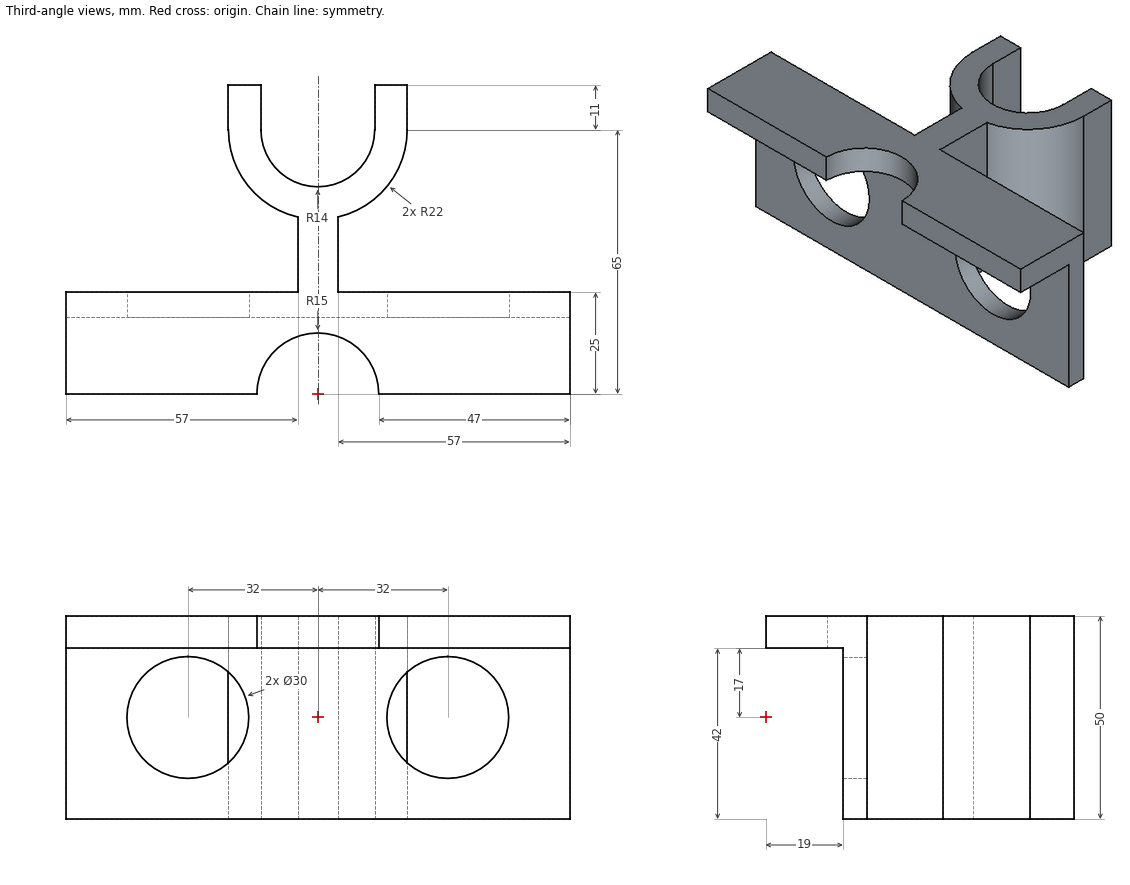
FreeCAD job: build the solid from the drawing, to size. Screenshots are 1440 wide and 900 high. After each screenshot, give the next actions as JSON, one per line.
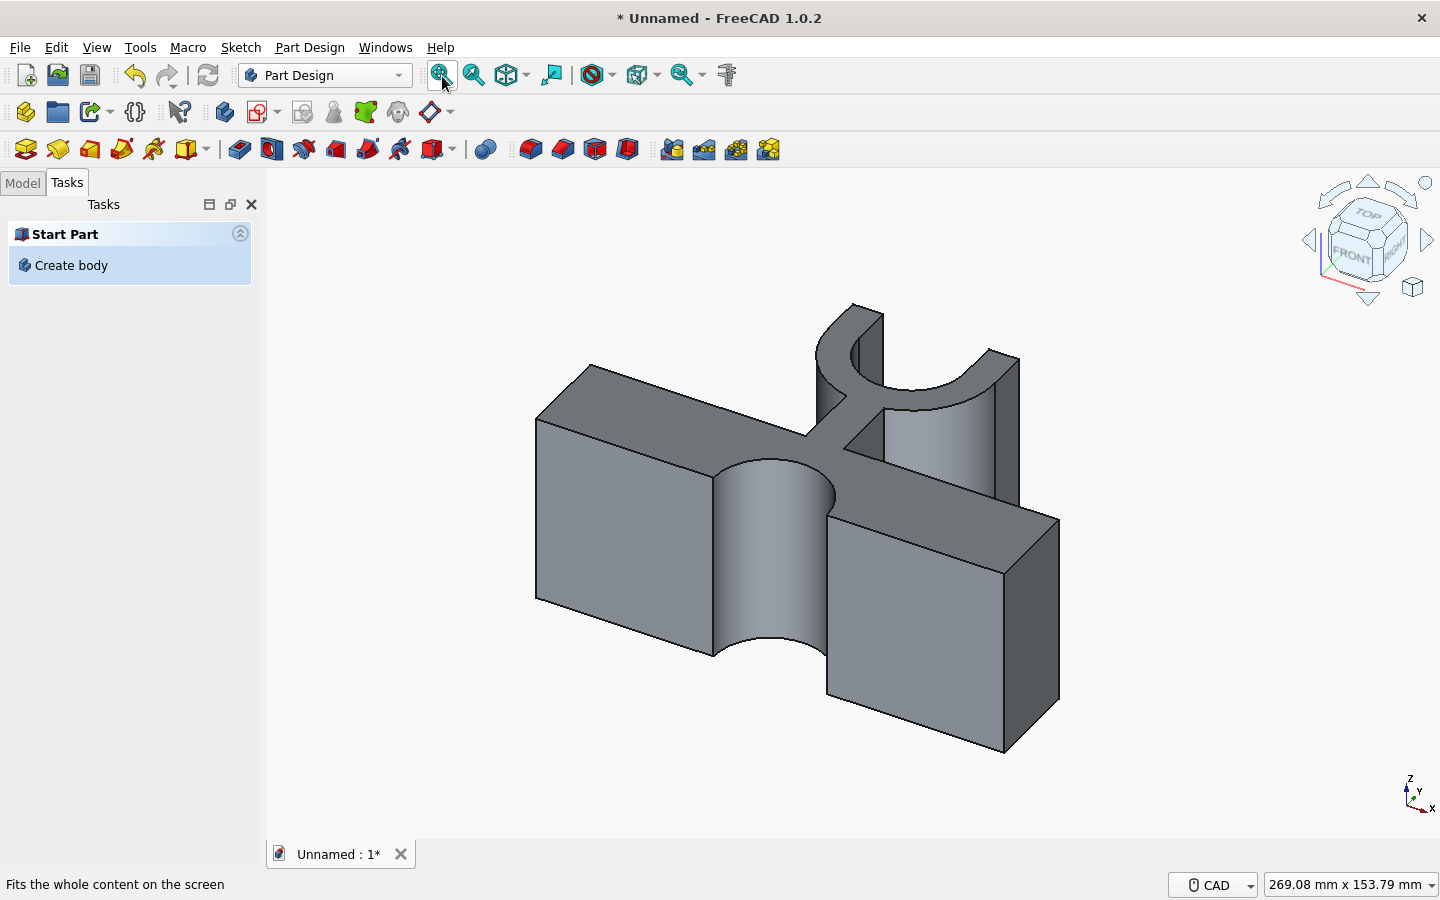
{"action": "left_click", "coordinate": [1032, 610]}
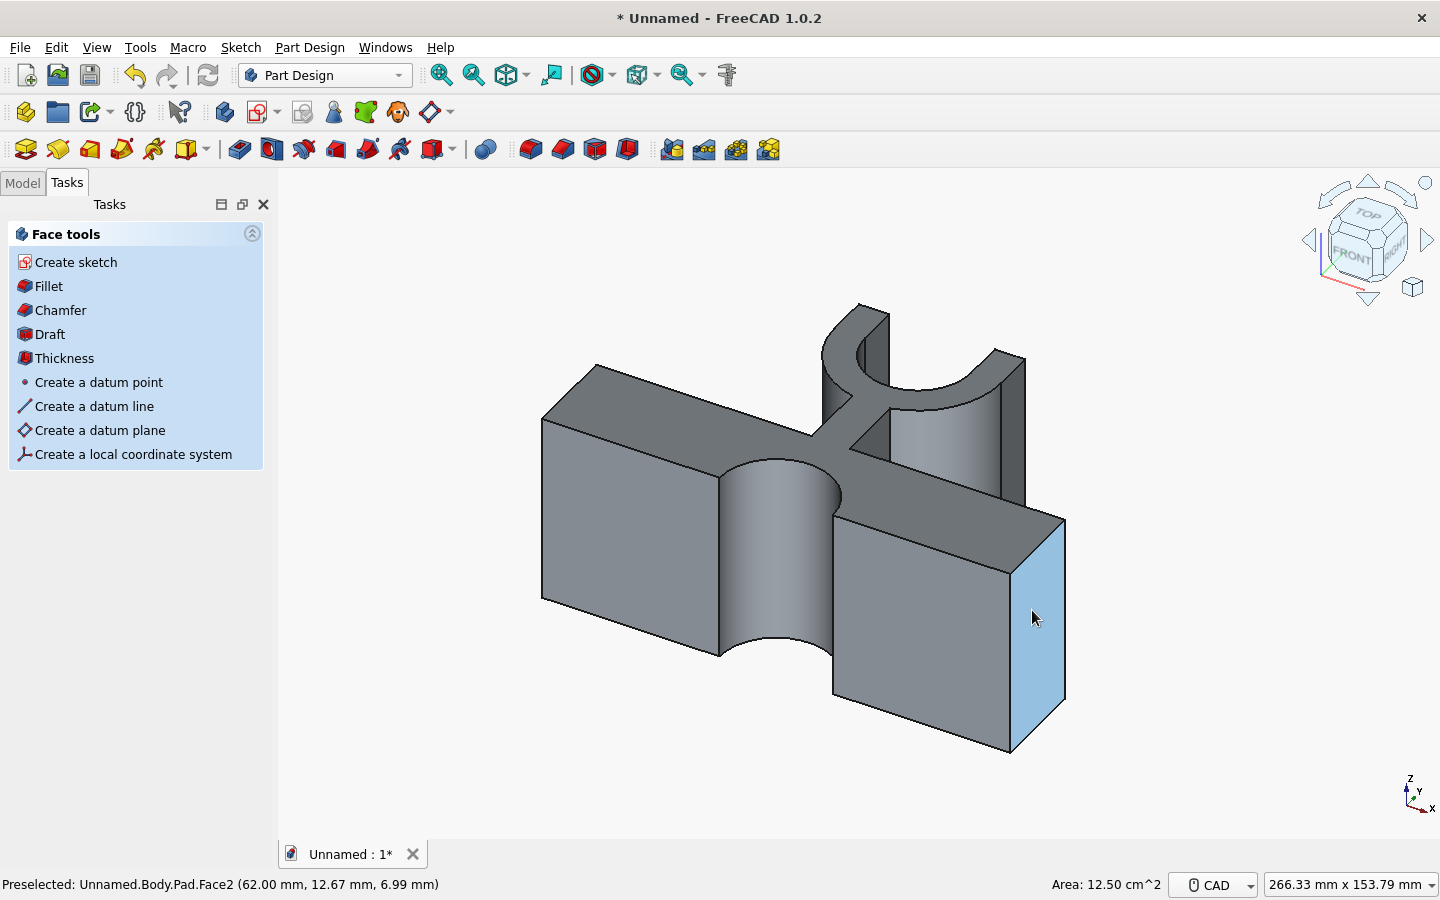
{"action": "left_click", "coordinate": [258, 112]}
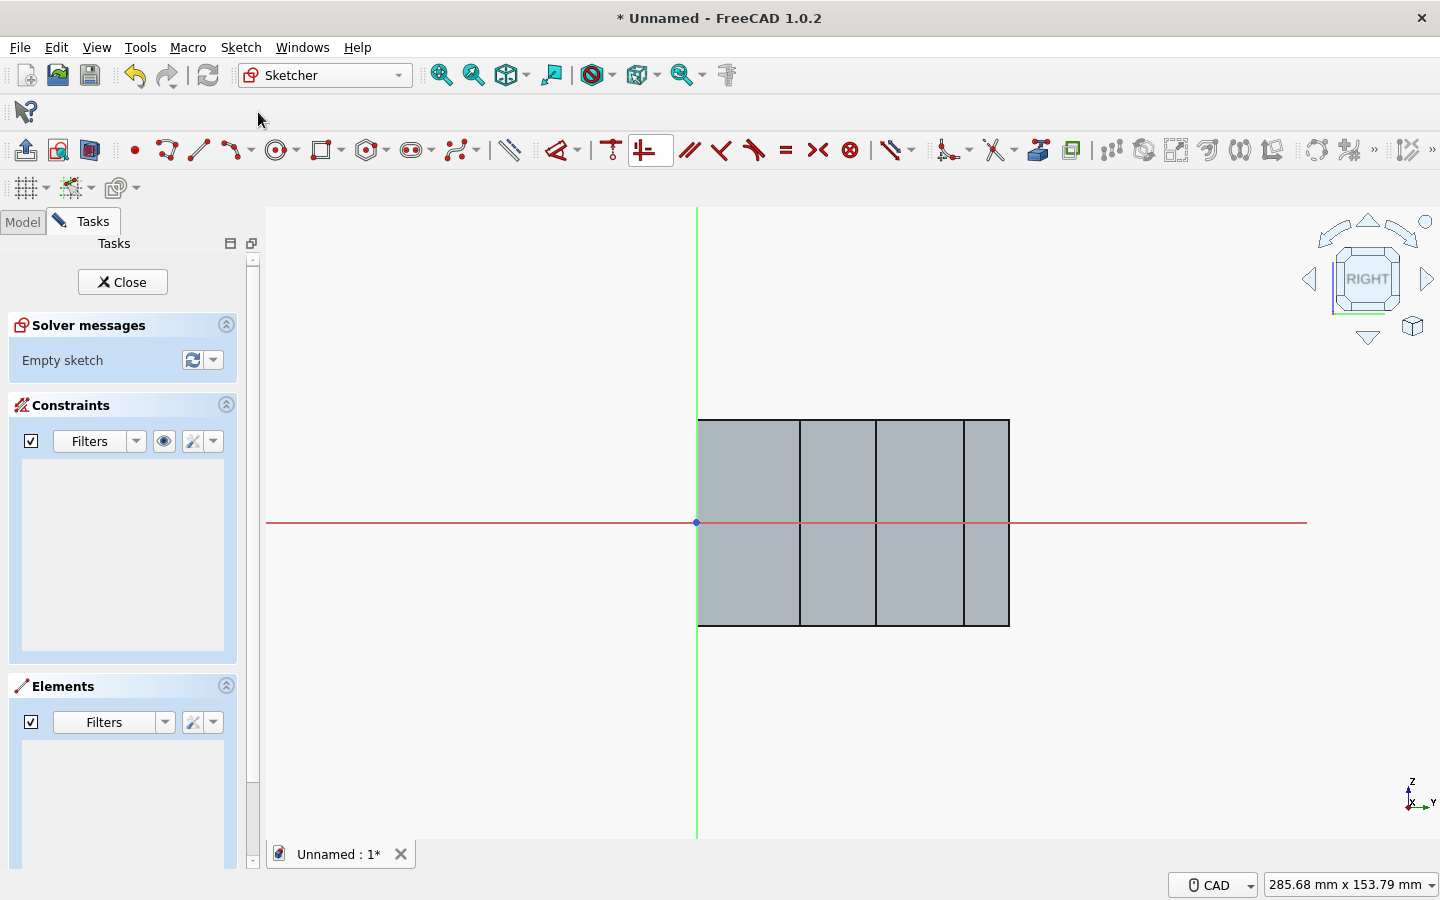
{"action": "scroll", "coordinate": [696, 553], "scroll_direction": "up", "scroll_amount": 4}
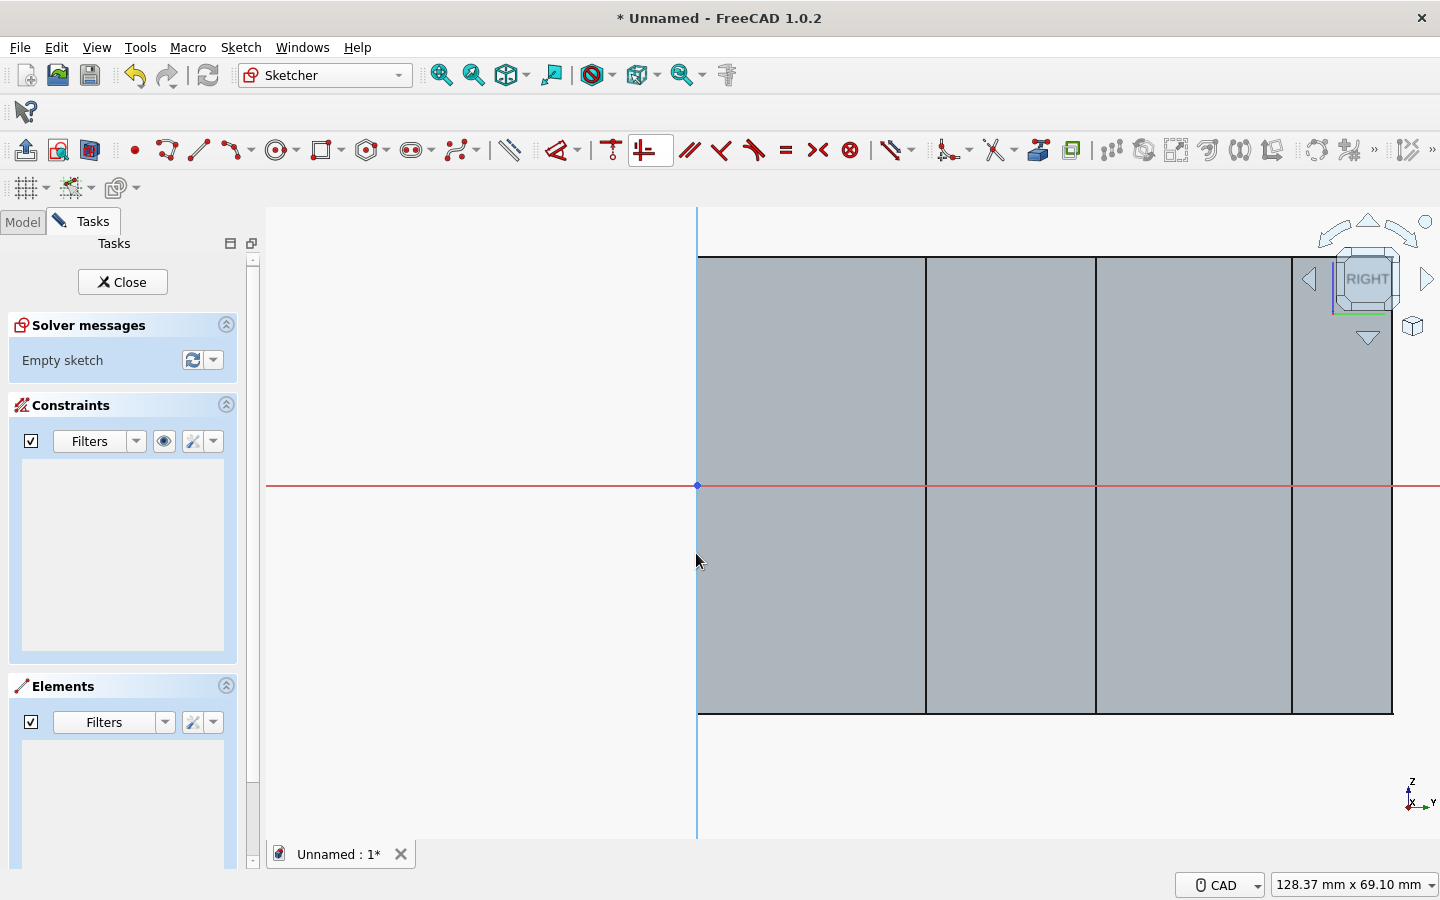
{"action": "left_click", "coordinate": [322, 150]}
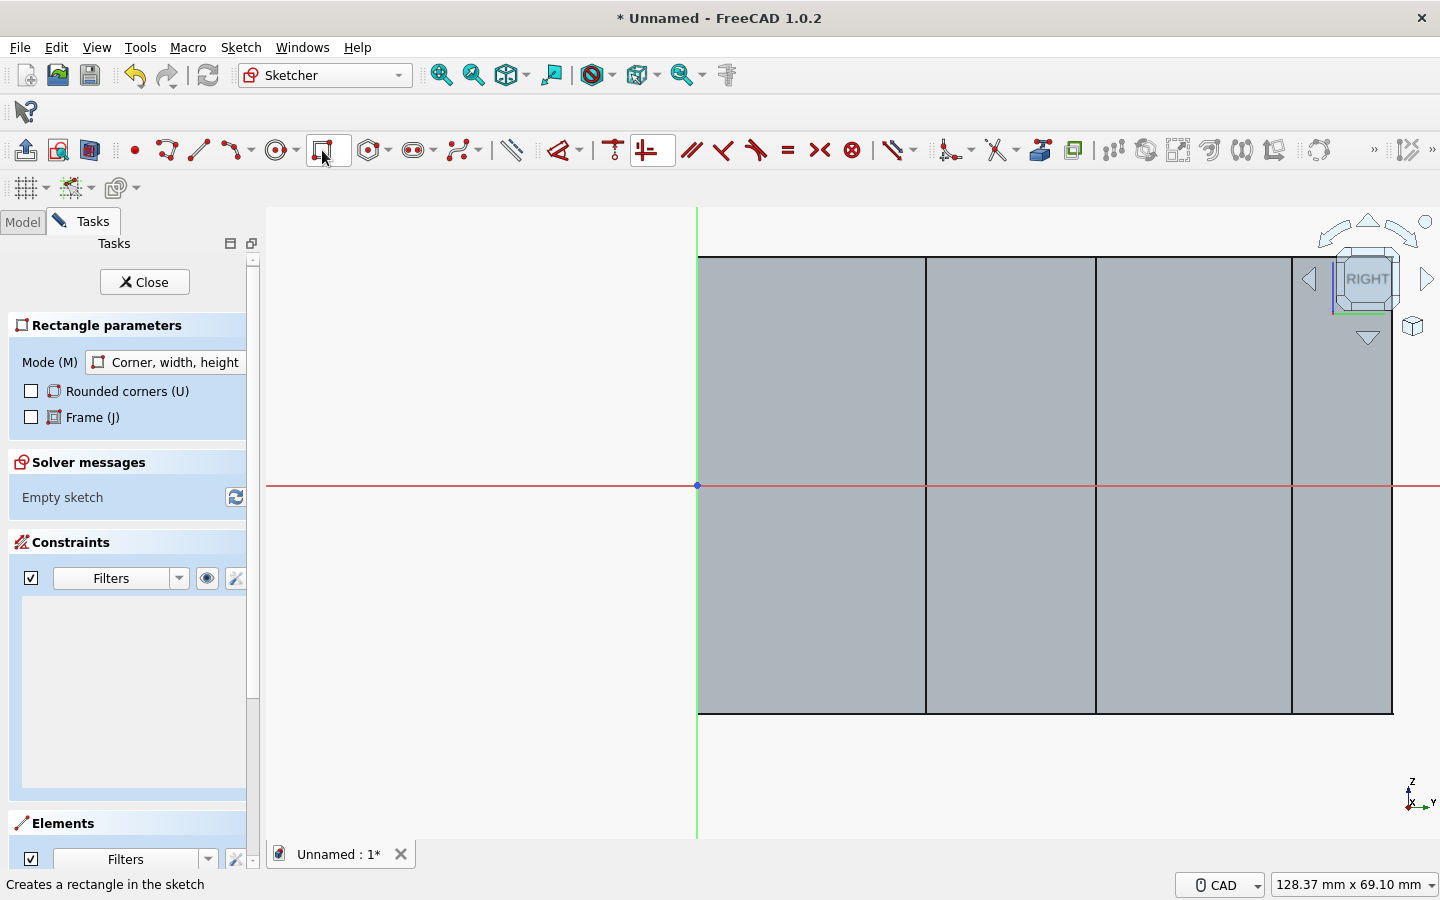
{"action": "left_click", "coordinate": [697, 330]}
{"action": "left_click", "coordinate": [871, 714]}
{"action": "key", "text": "Escape"}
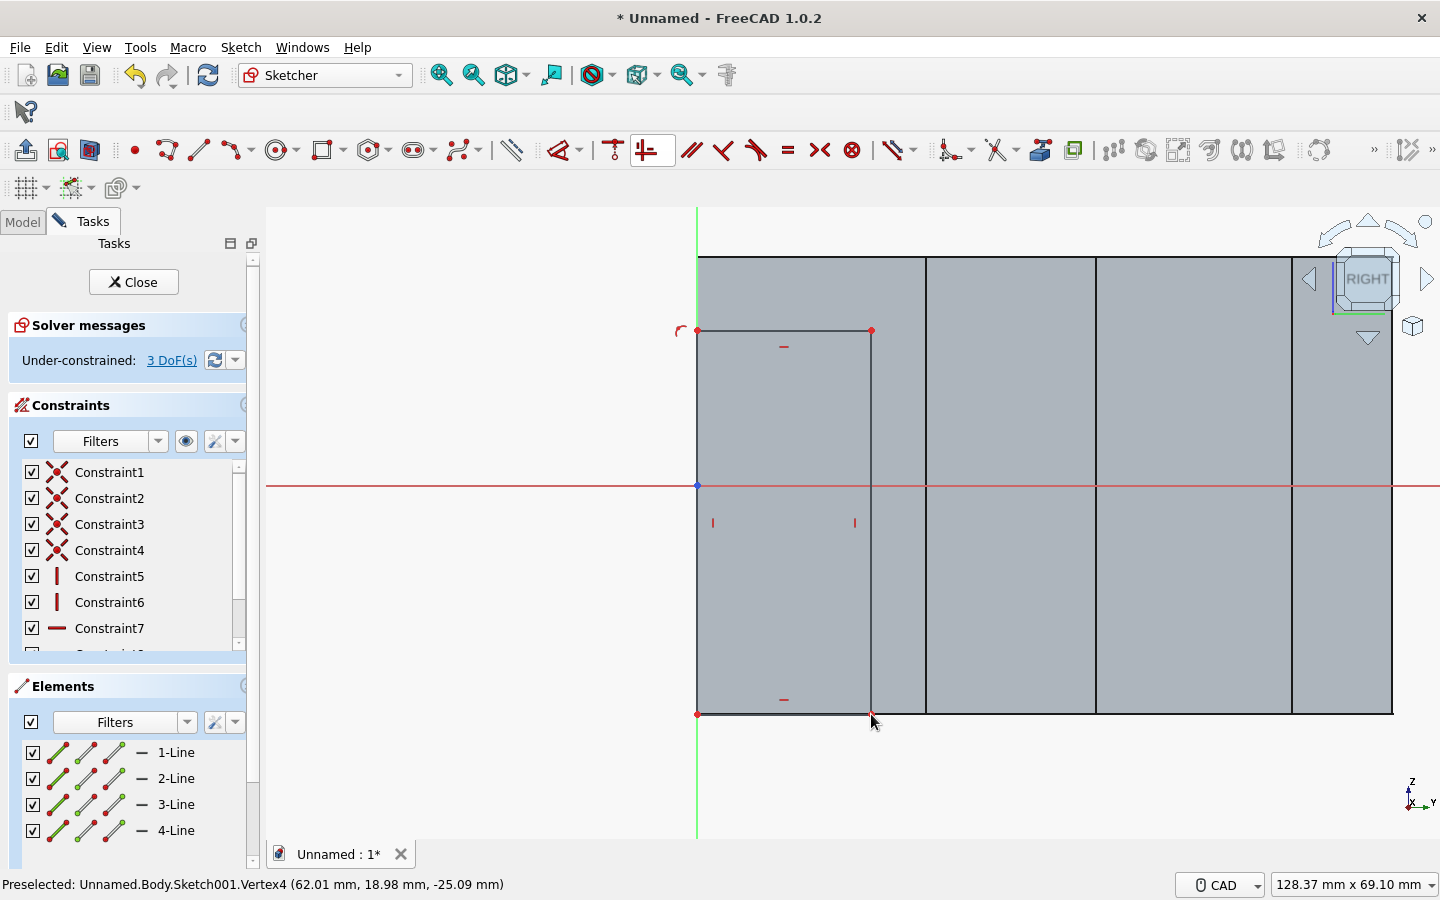
{"action": "left_click", "coordinate": [558, 150]}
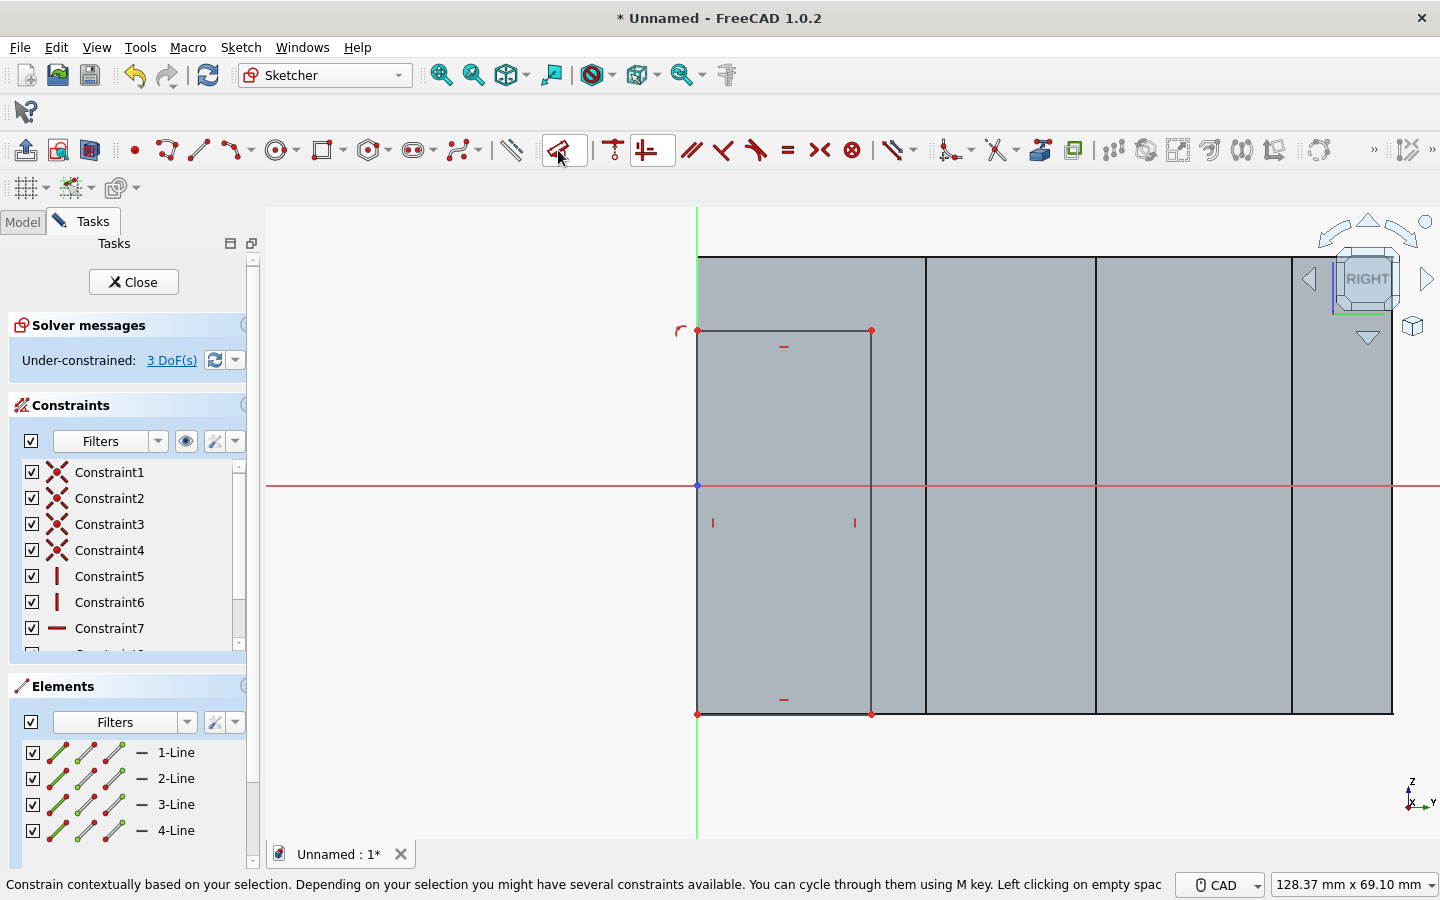
{"action": "left_click", "coordinate": [697, 446]}
{"action": "left_click", "coordinate": [663, 523]}